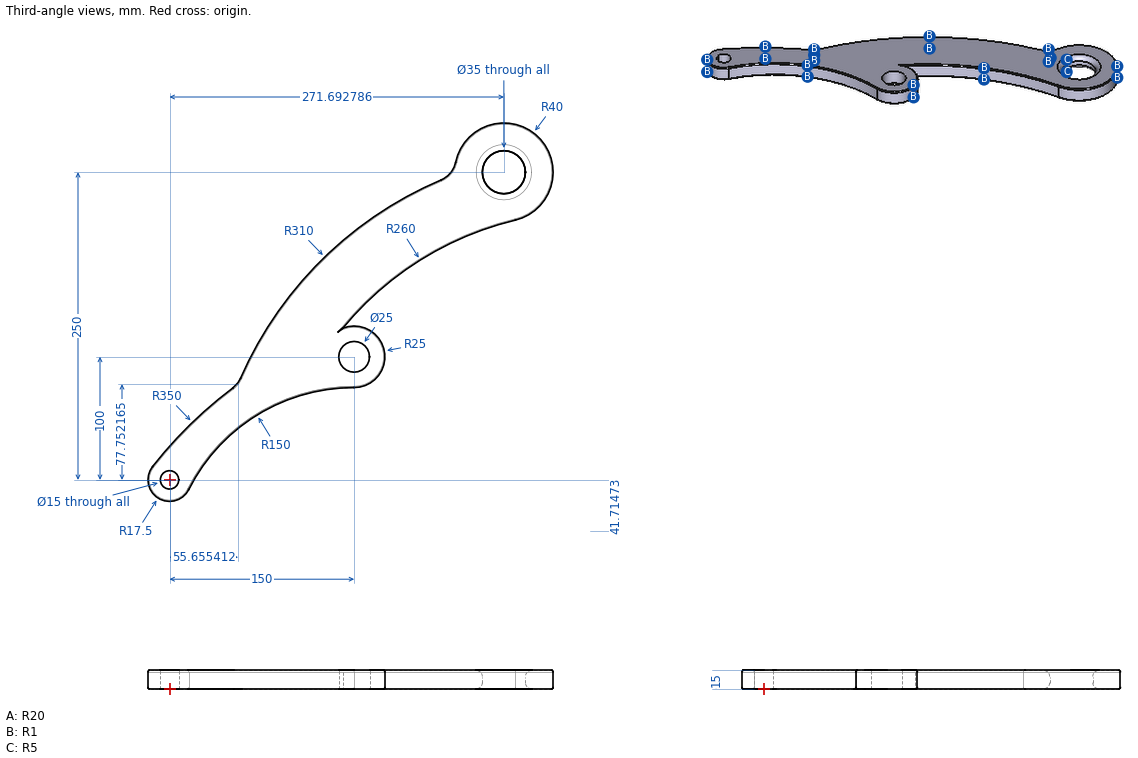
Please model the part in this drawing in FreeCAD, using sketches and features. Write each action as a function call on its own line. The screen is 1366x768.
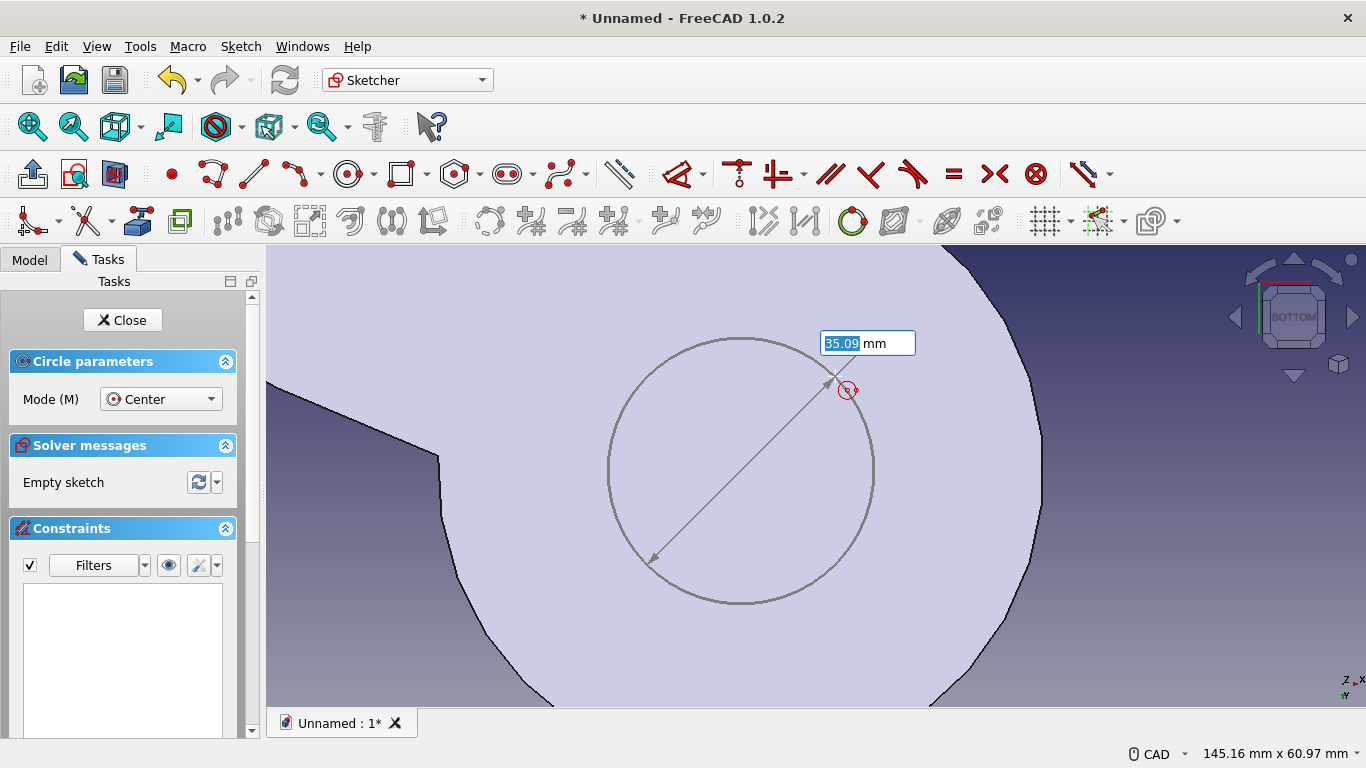
text(35)
key(Return)
key(Escape)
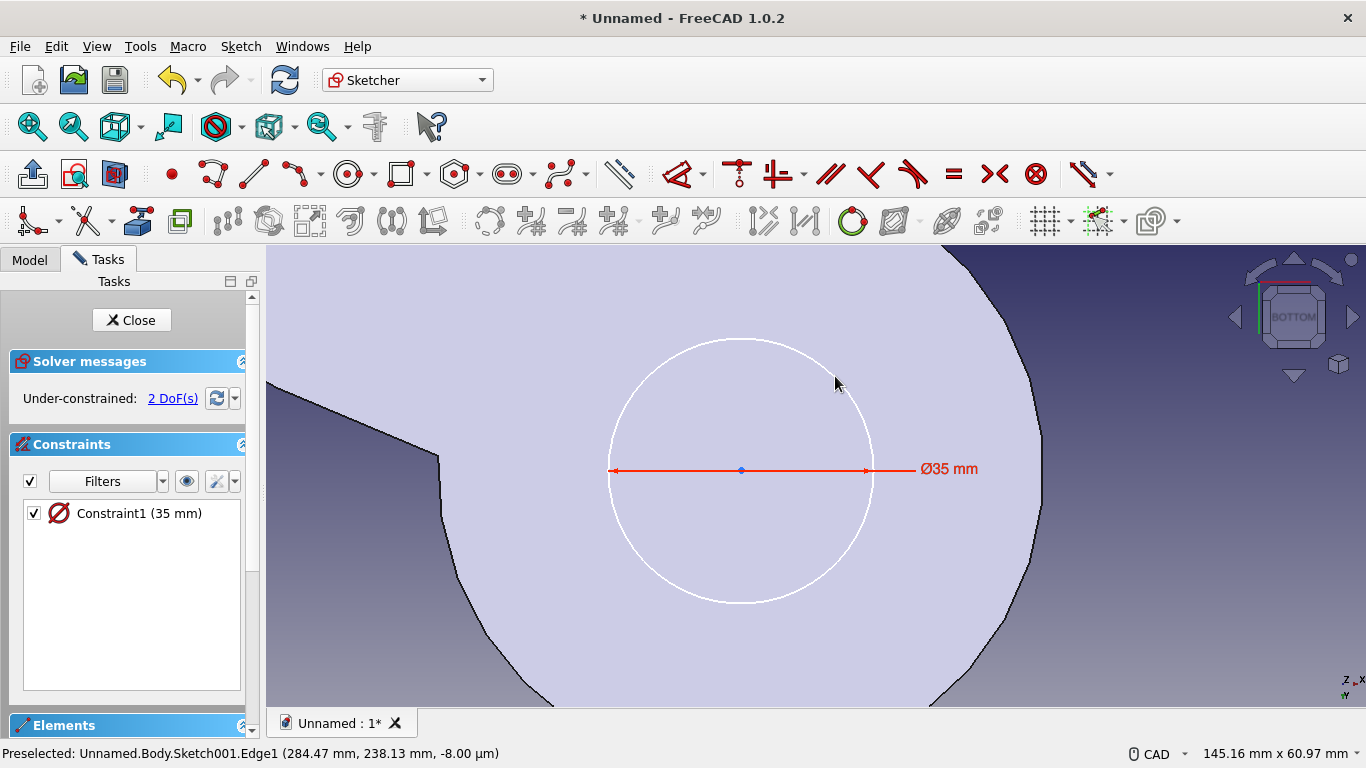
click(676, 174)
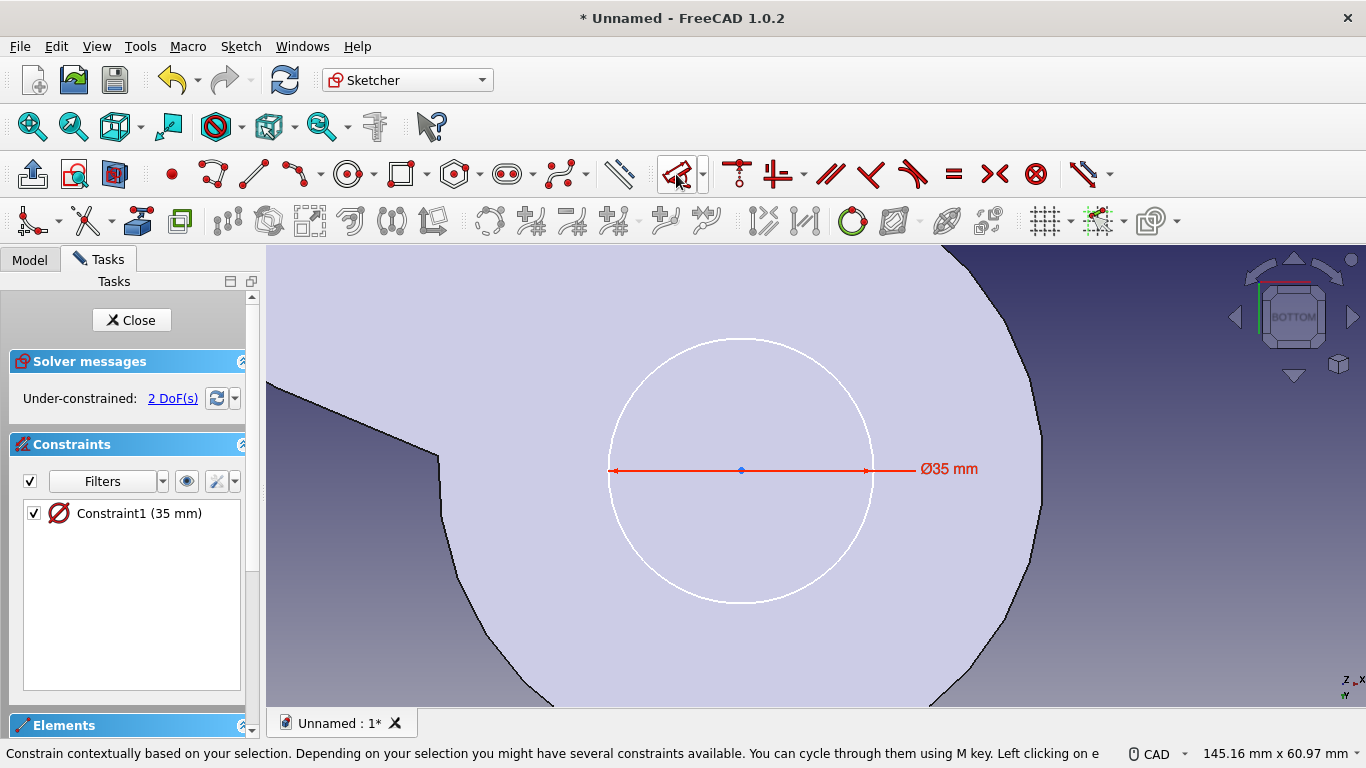
click(741, 471)
click(775, 372)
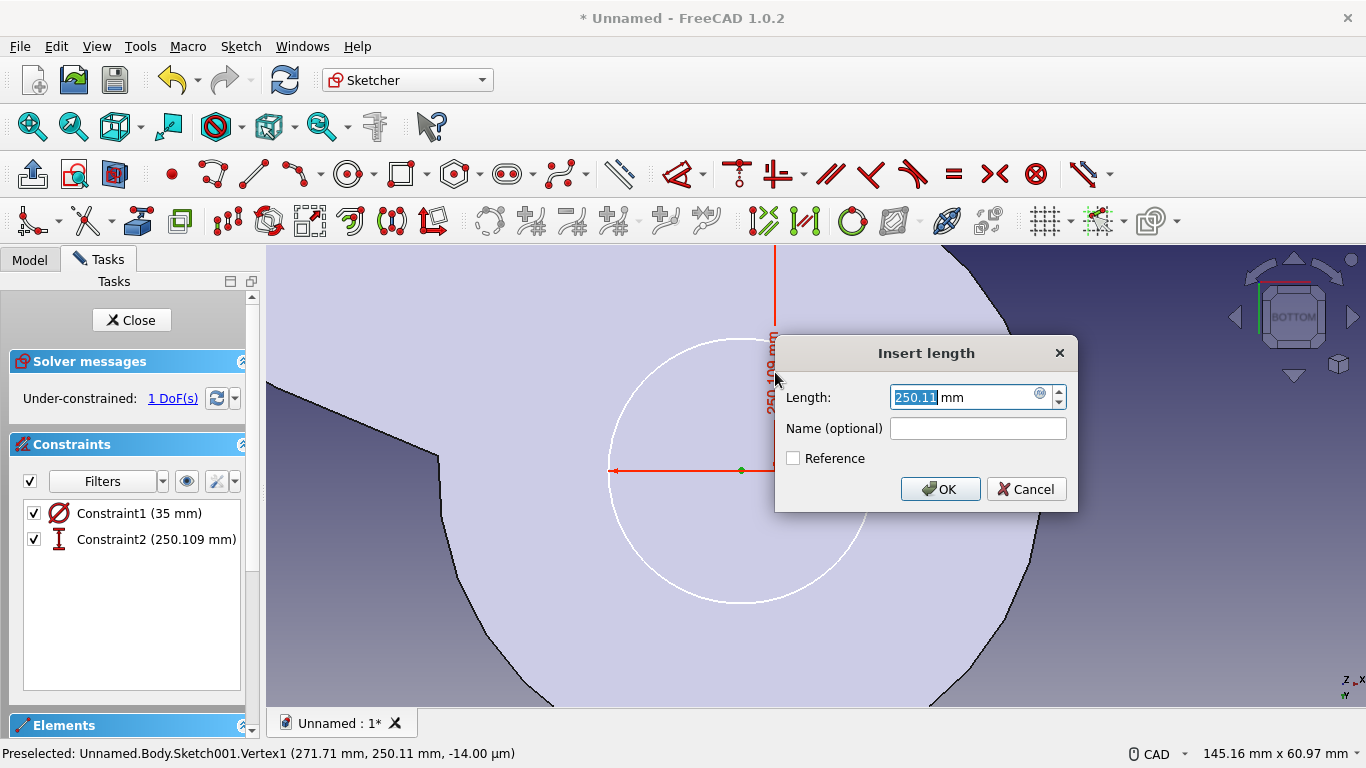
text(250)
key(Return)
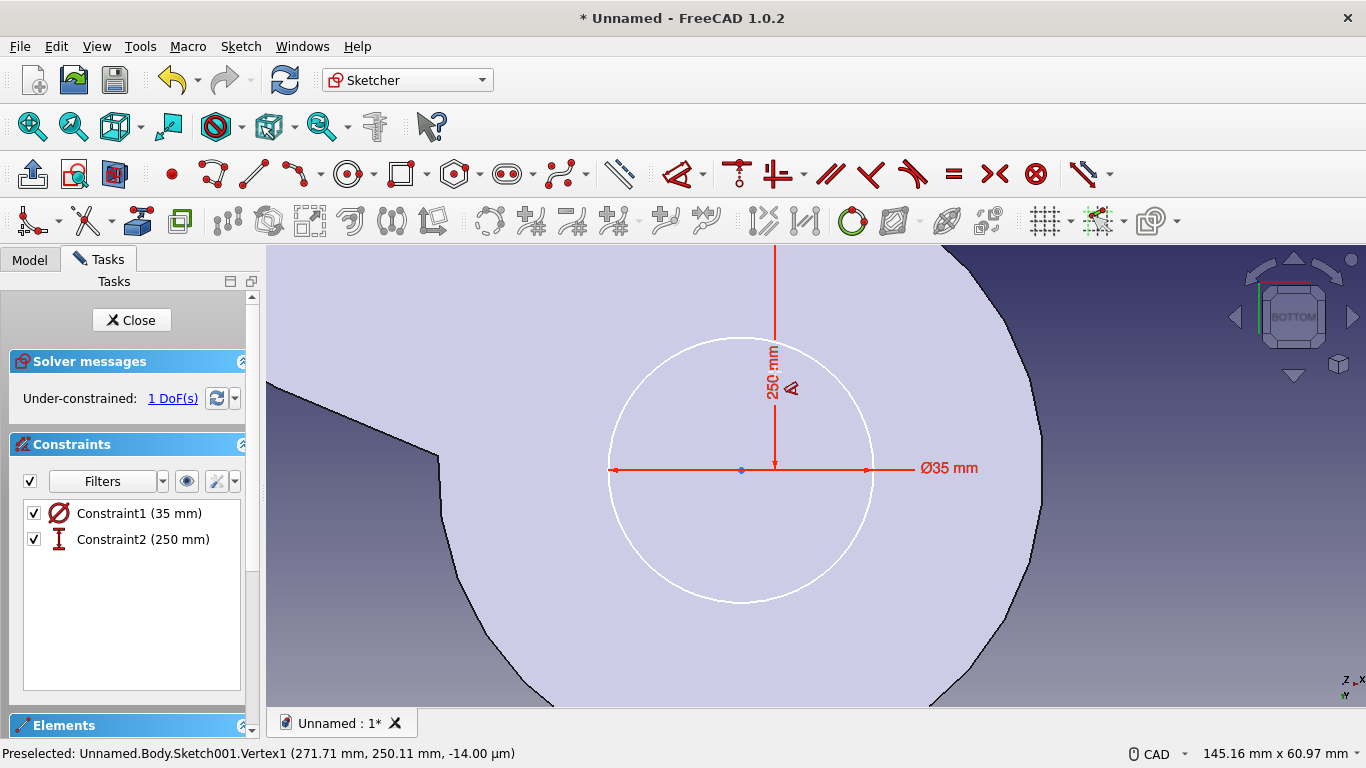
click(741, 470)
click(517, 504)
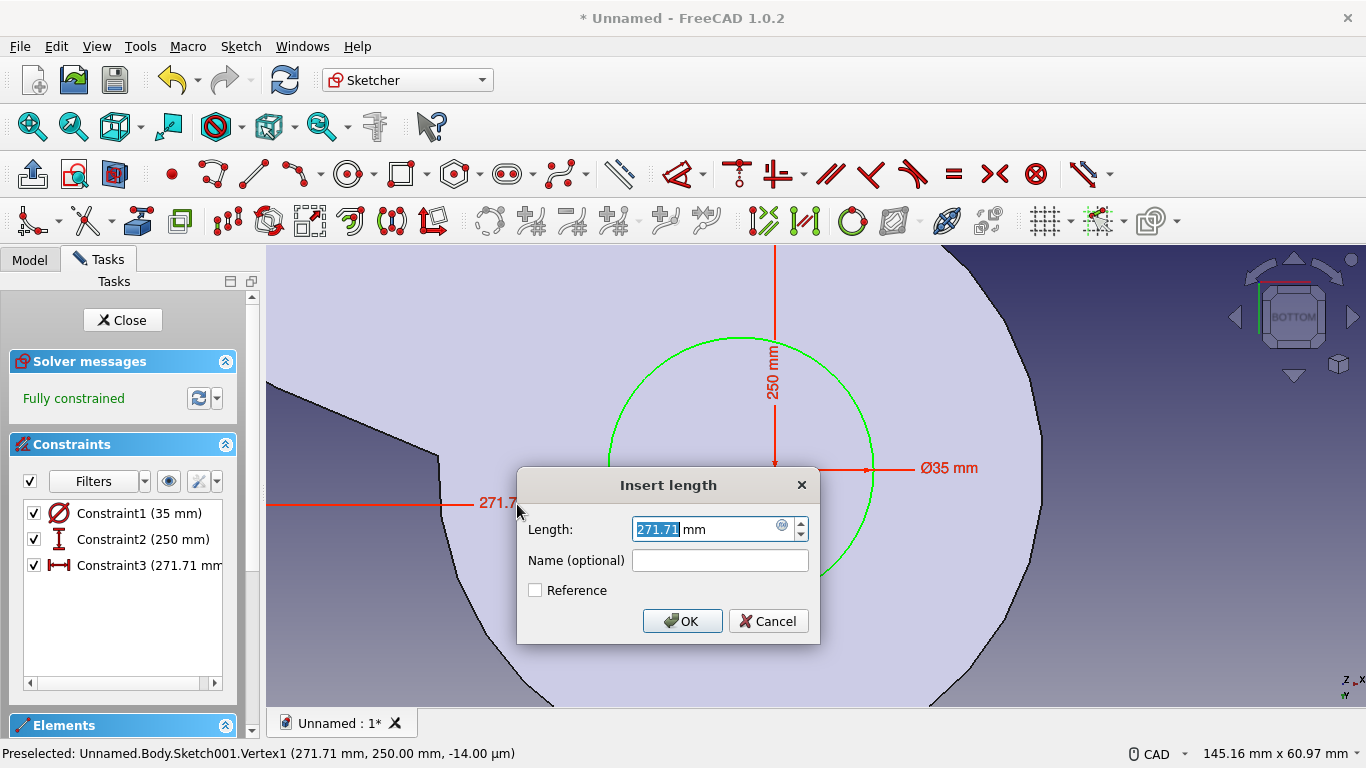
text(271.692786)
key(Return)
key(Escape)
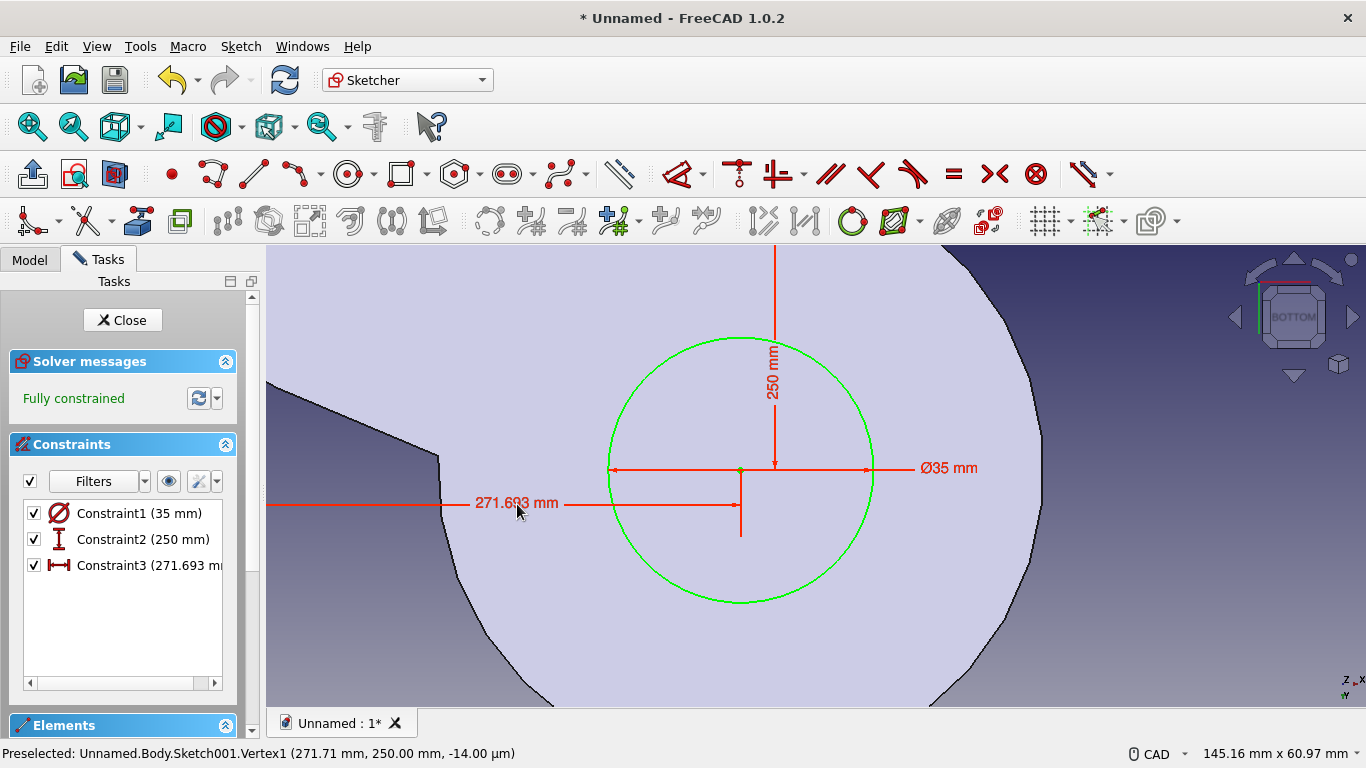
click(123, 320)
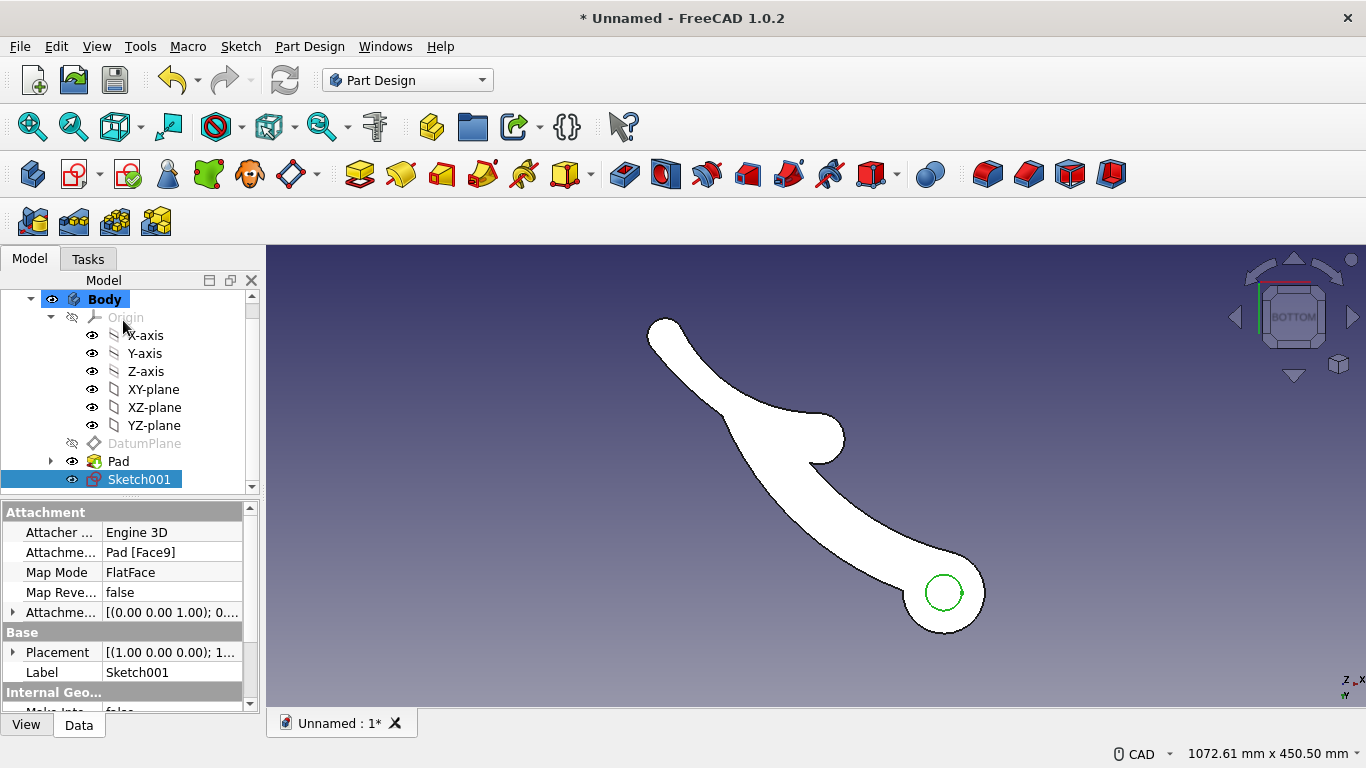
click(666, 174)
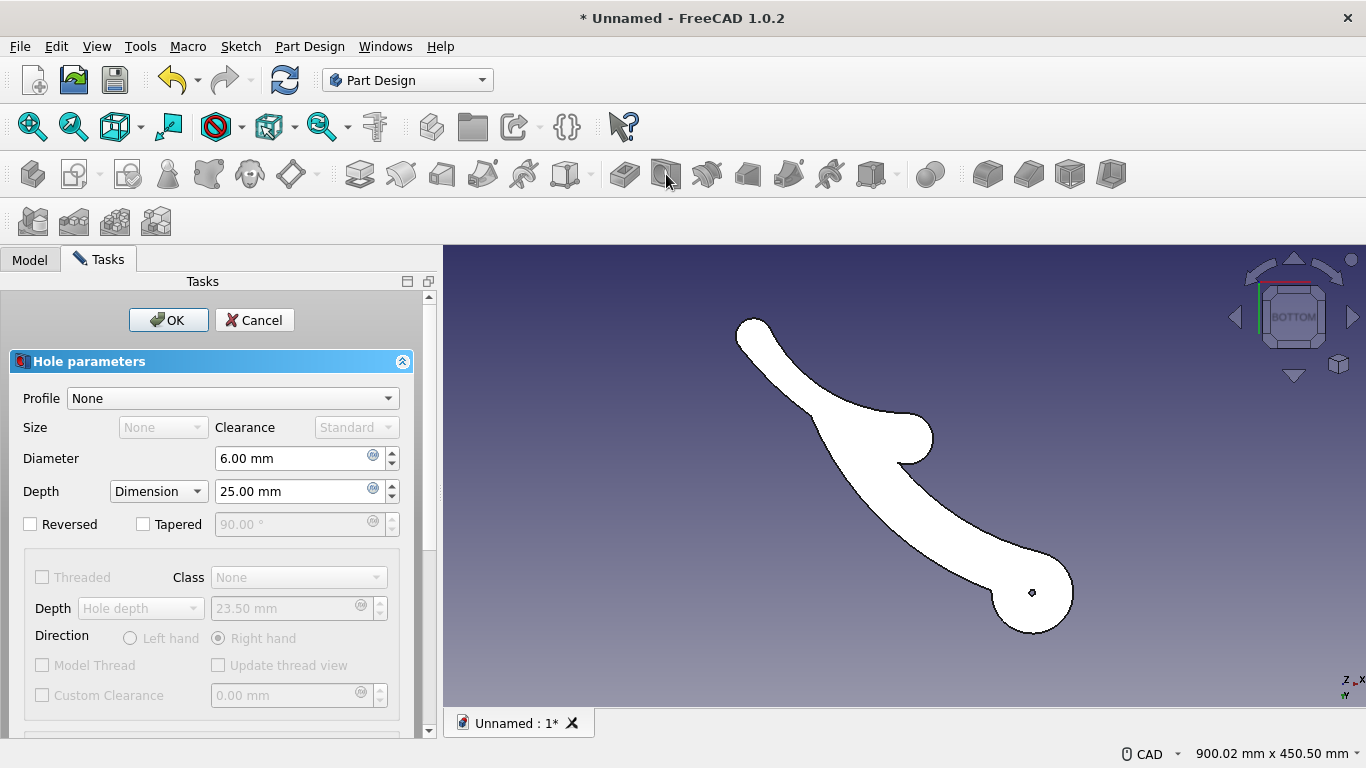
triple_click(300, 458)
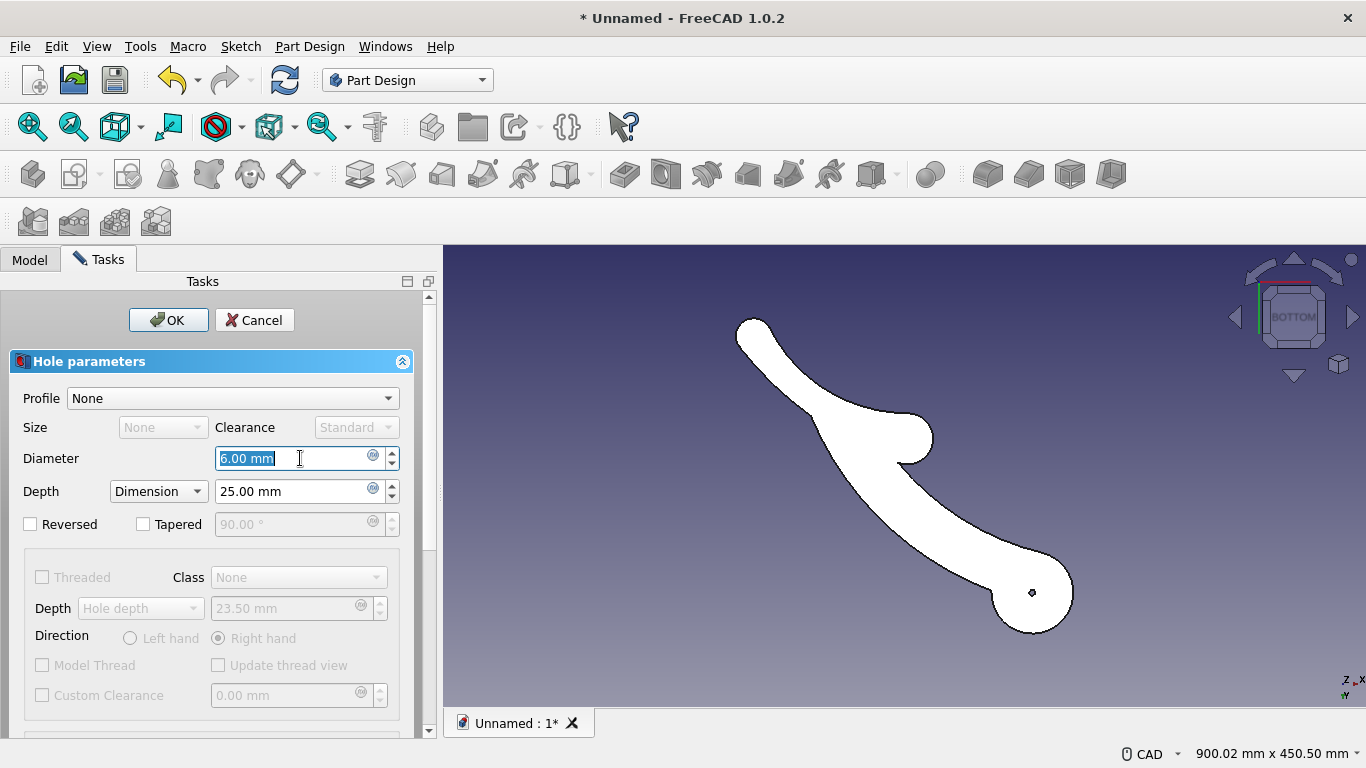
text(35)
key(Tab)